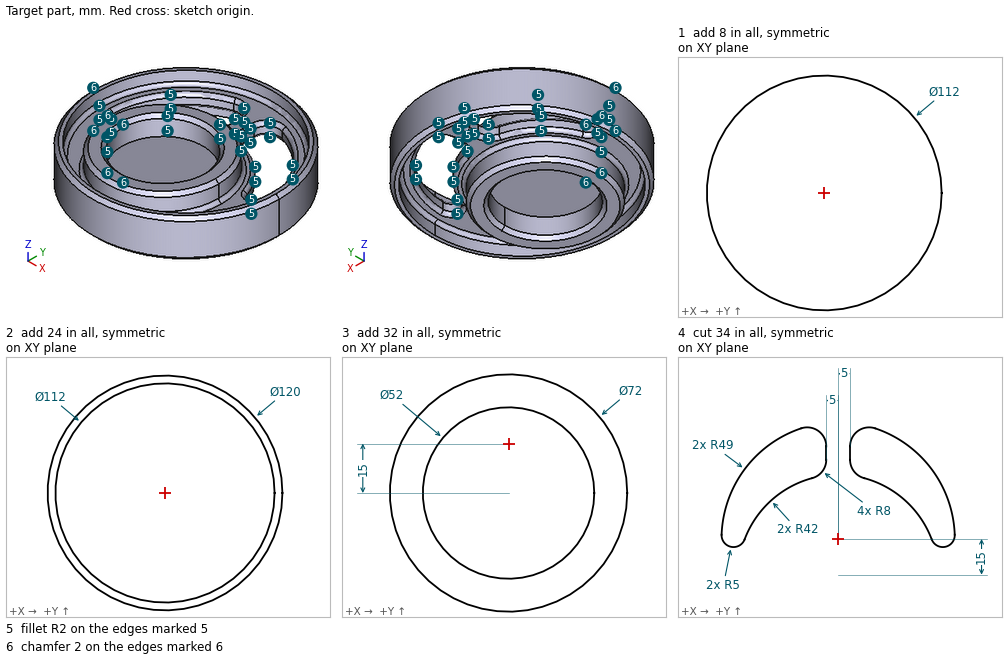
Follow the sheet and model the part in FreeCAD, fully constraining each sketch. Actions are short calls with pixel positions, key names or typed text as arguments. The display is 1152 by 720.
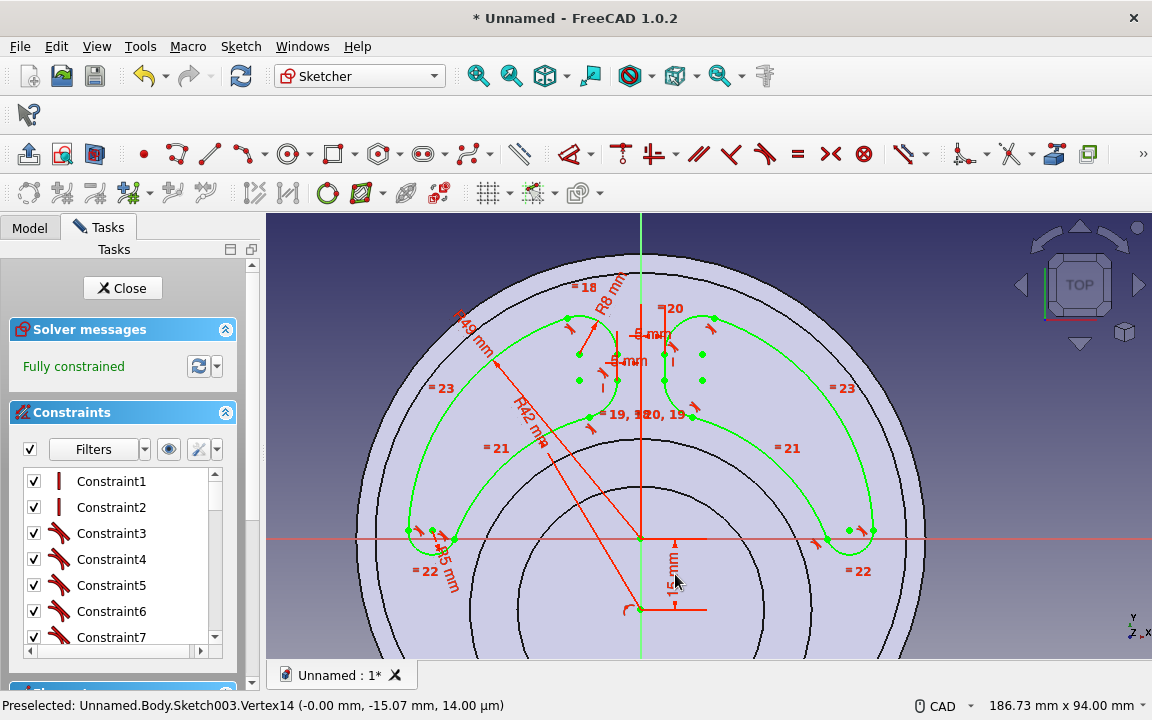
click(123, 288)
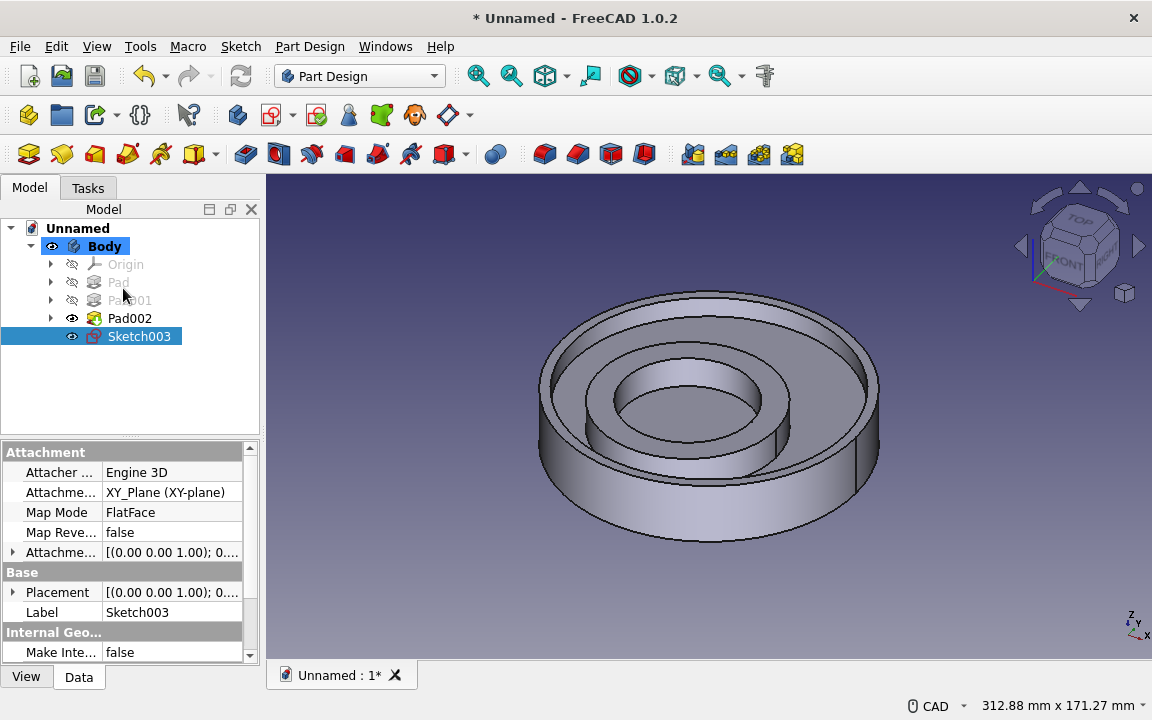
click(246, 154)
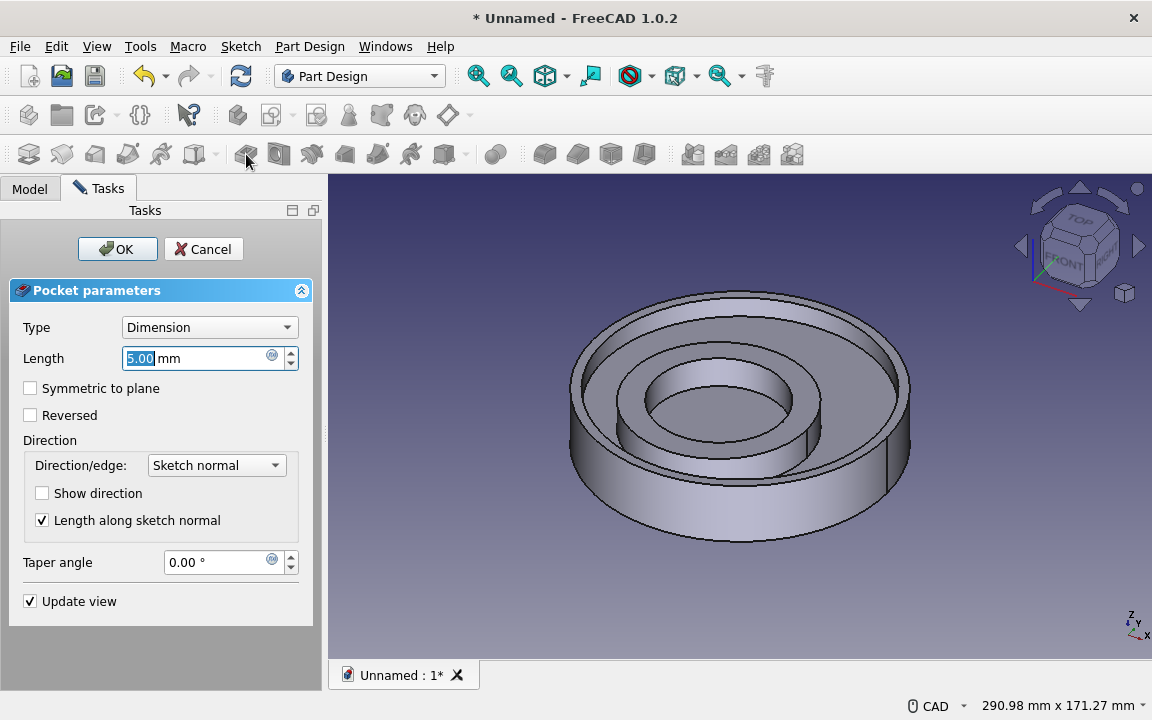
text(34)
key(Tab)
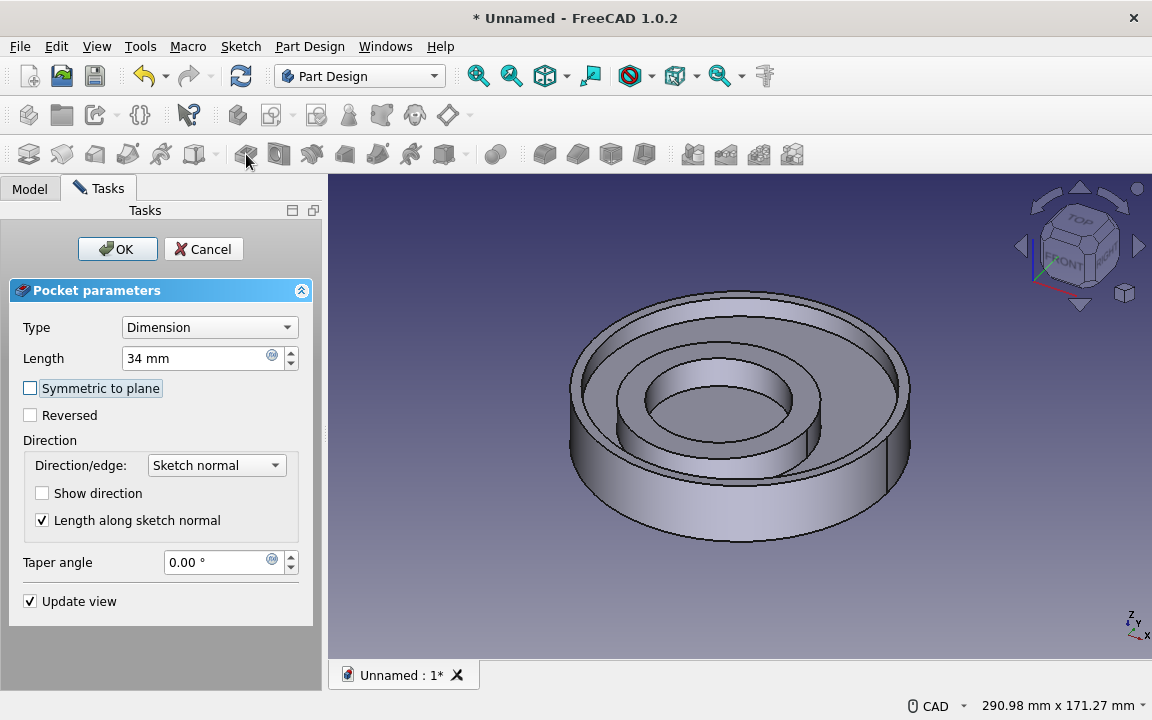
click(31, 388)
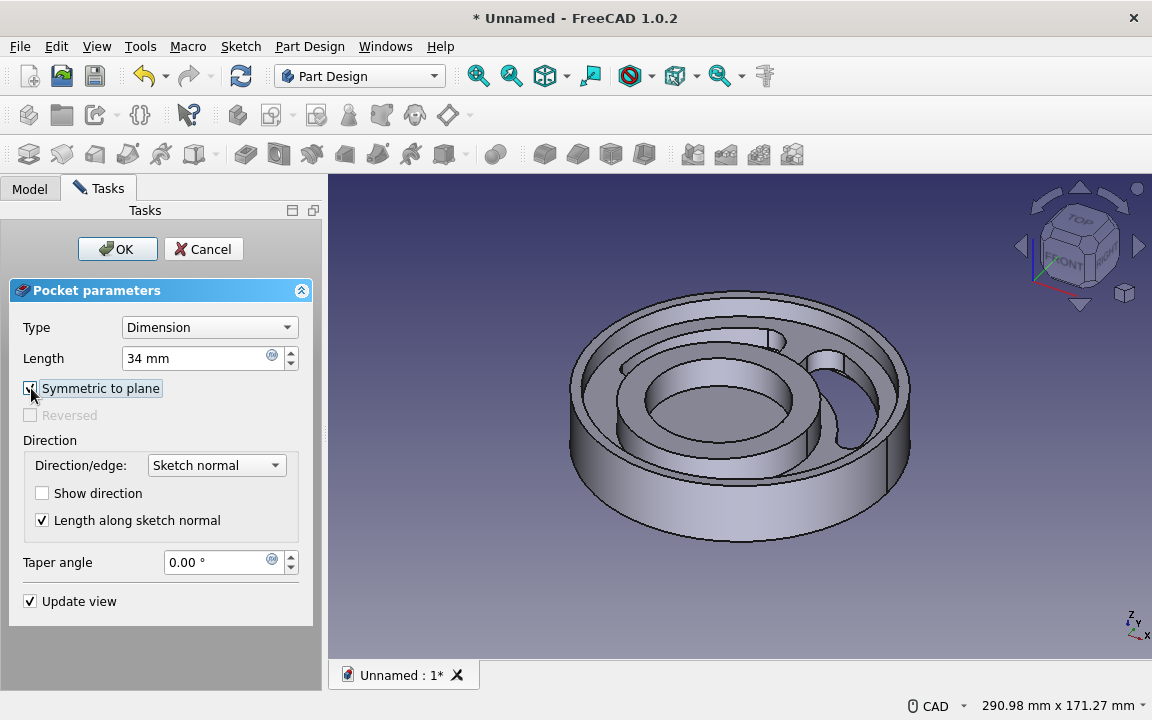
click(118, 249)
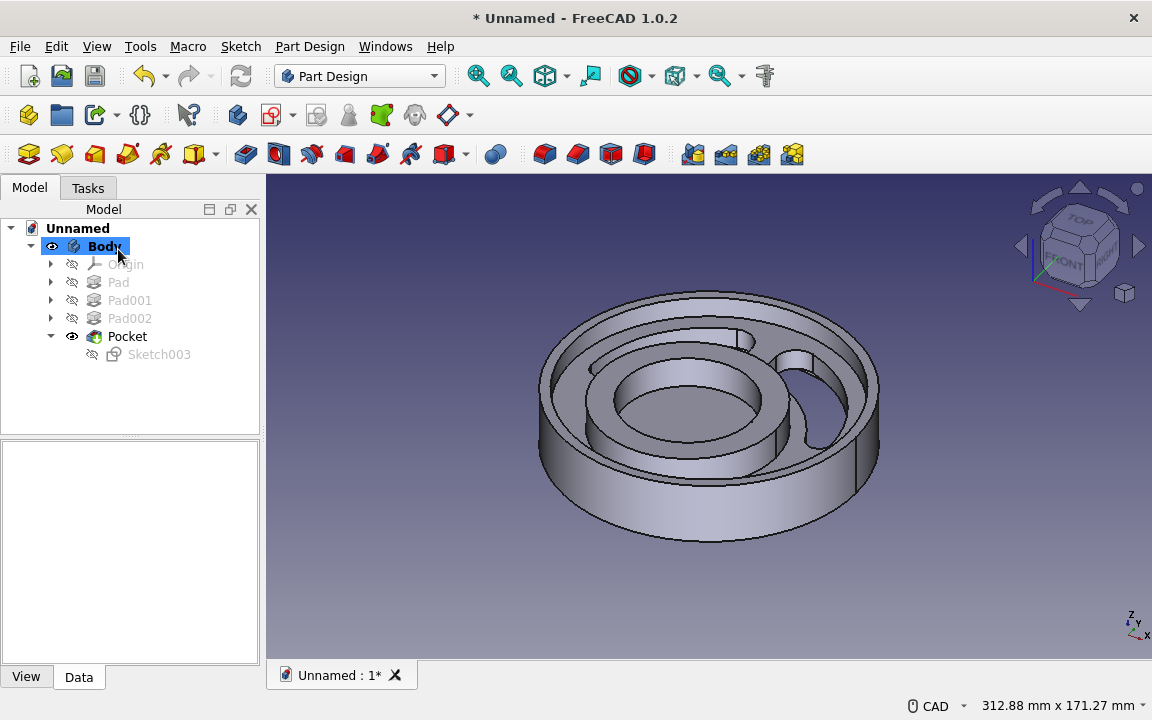
click(777, 339)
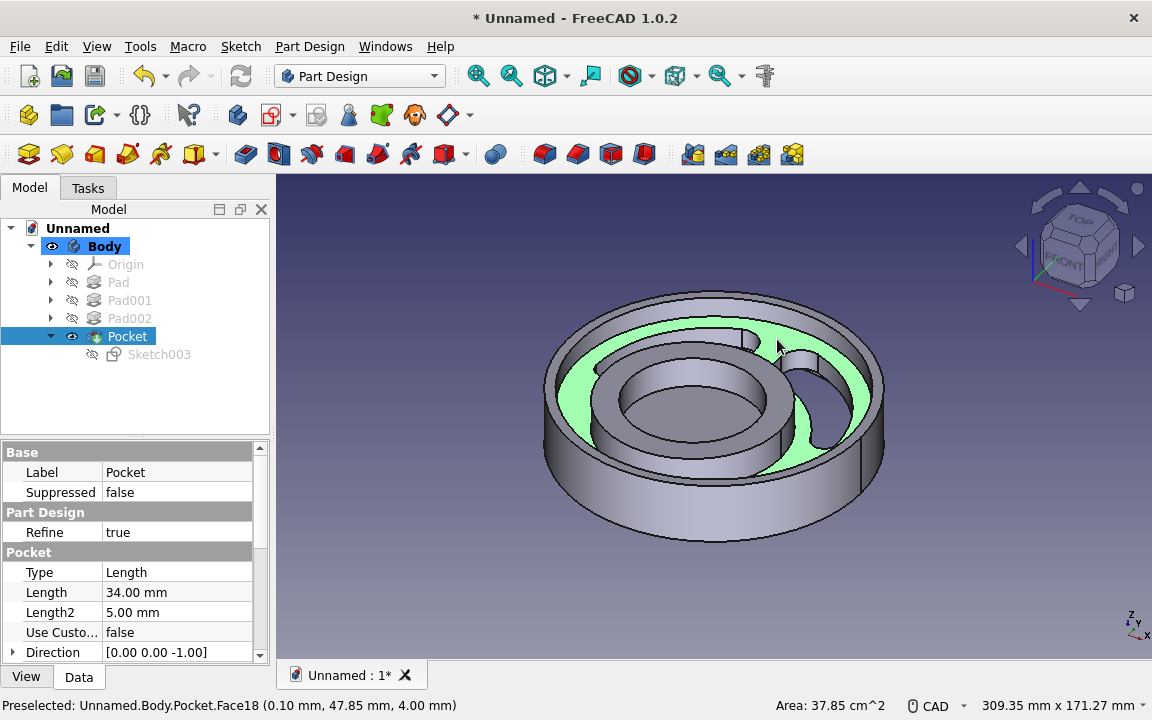
key(0)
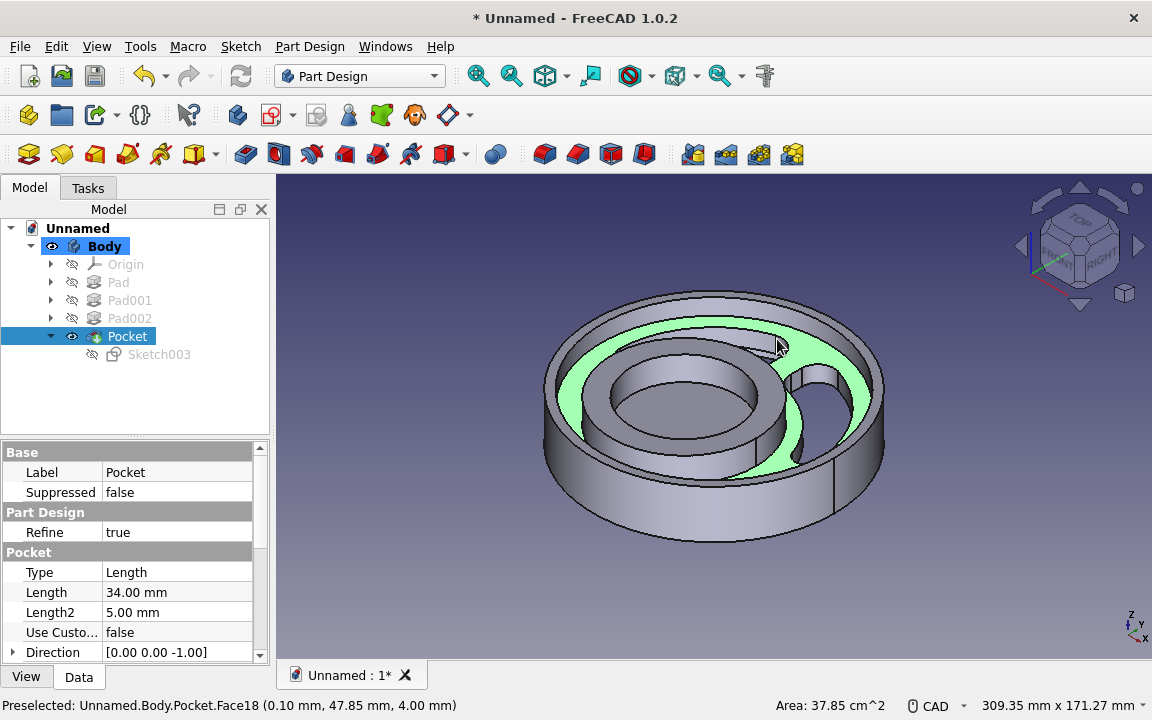
key(2)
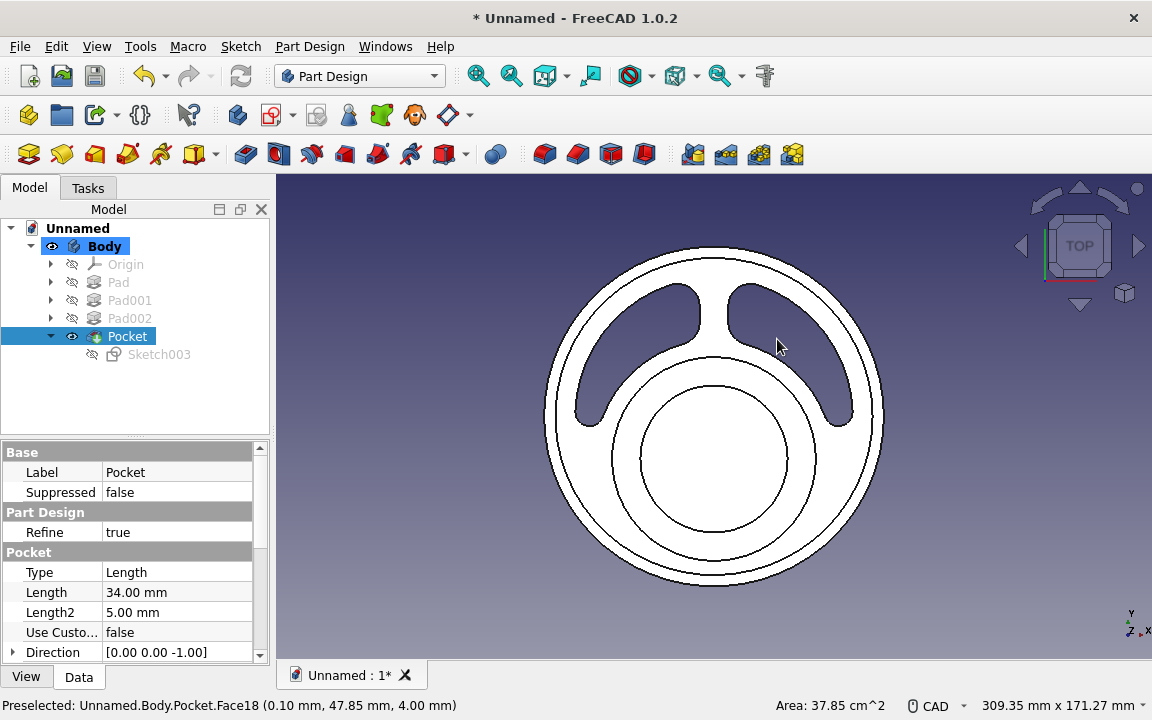
key(1)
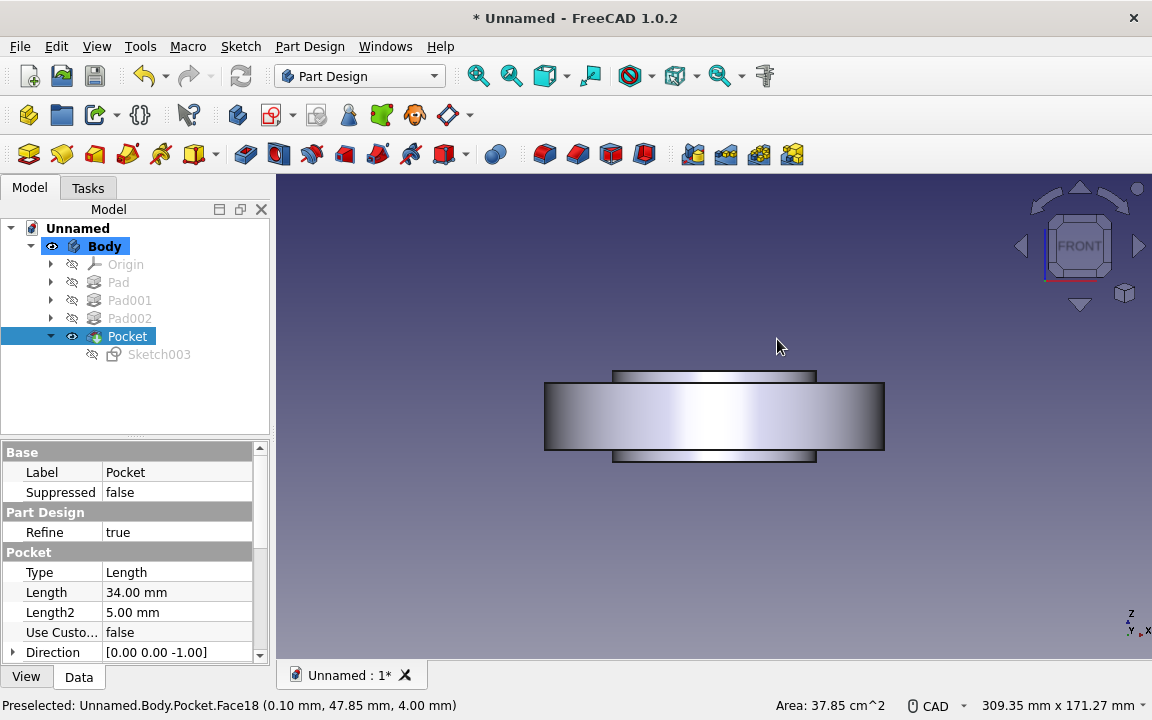
key(v)
key(f)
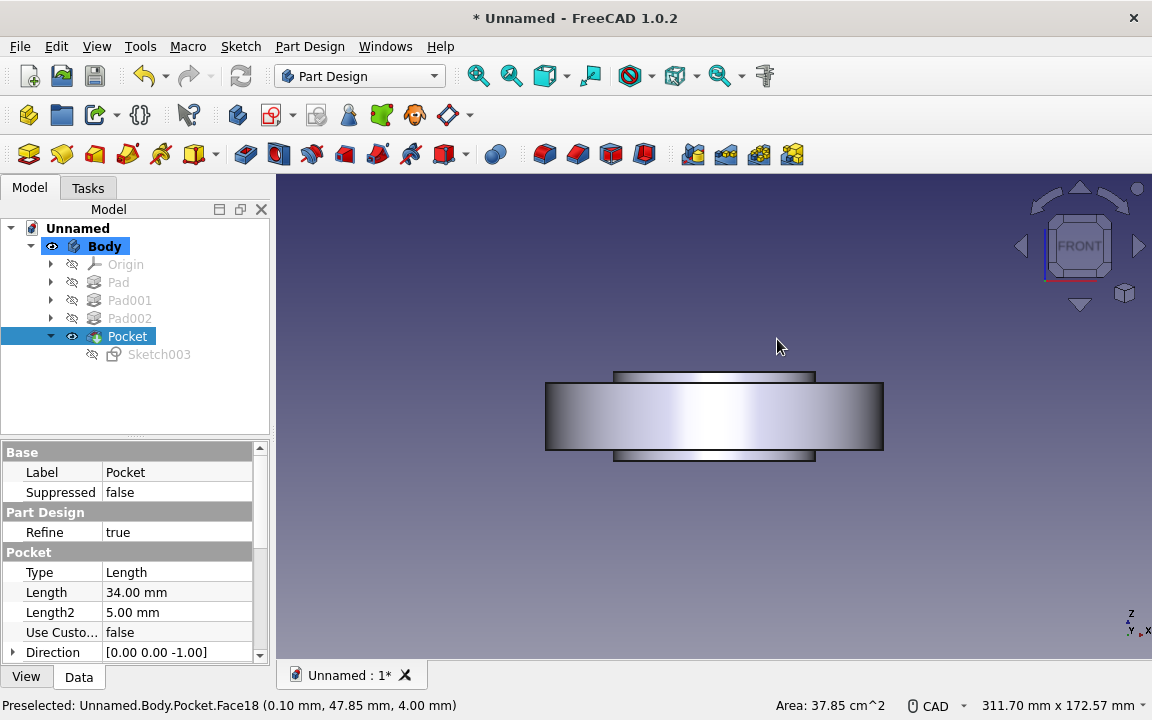
key(3)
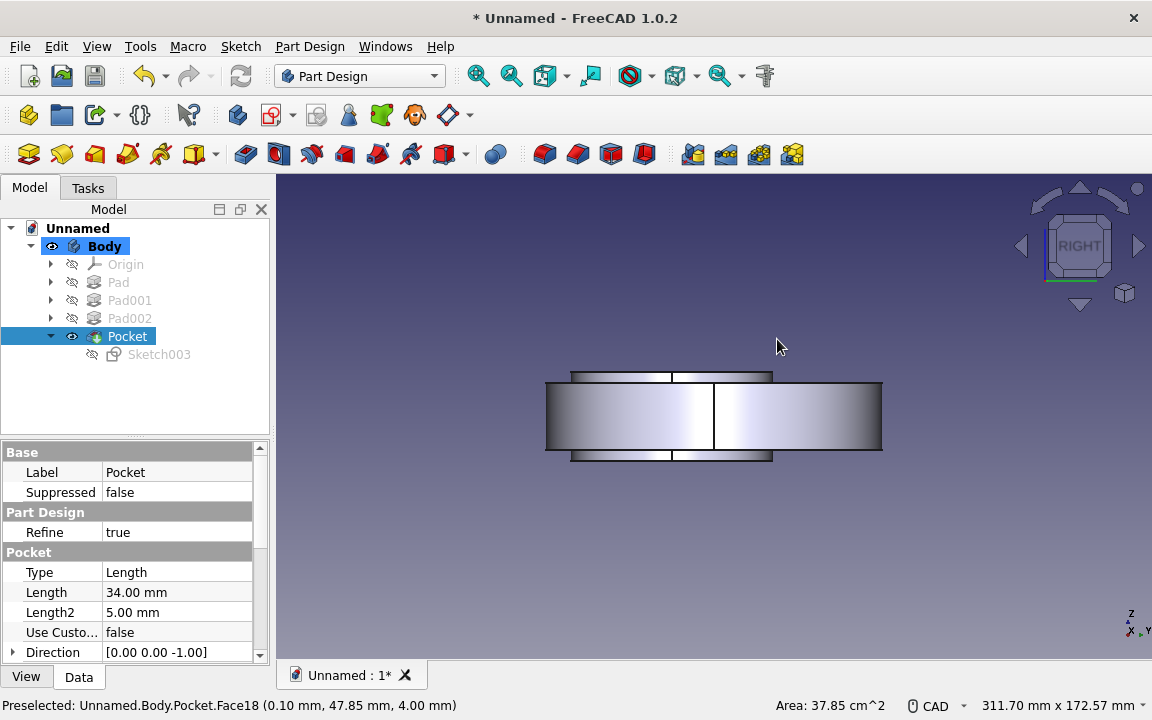
key(v)
key(f)